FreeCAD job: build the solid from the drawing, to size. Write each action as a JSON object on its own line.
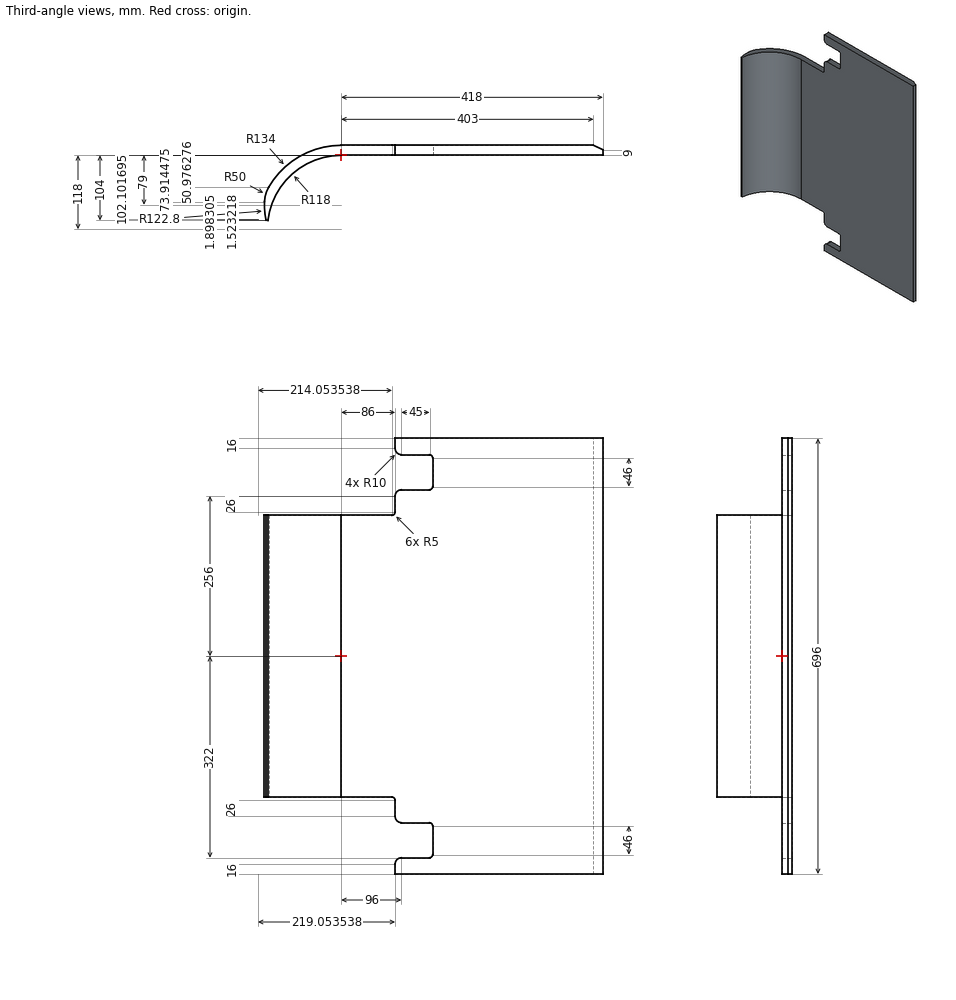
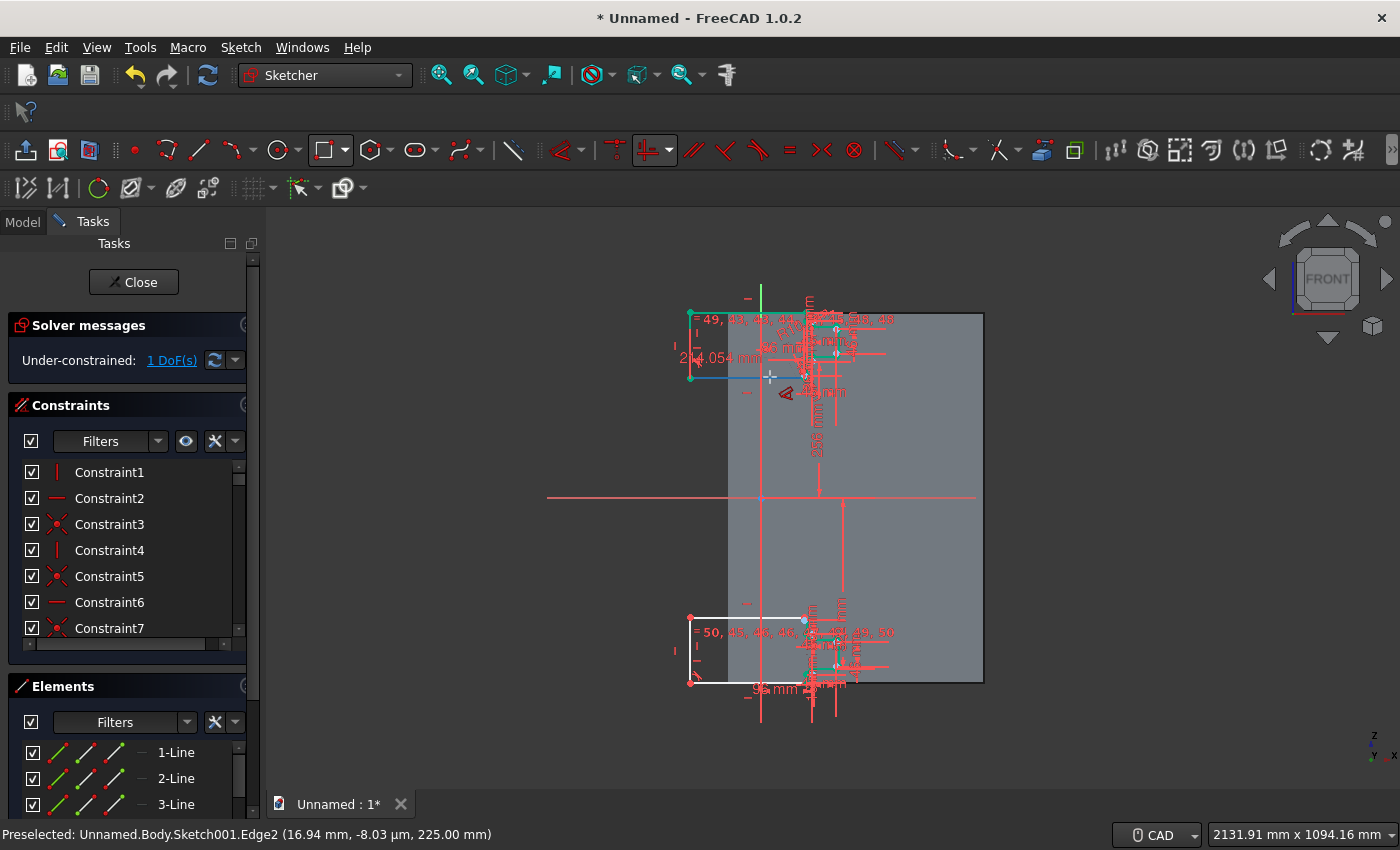
{"action": "scroll", "coordinate": [772, 683], "scroll_direction": "up", "scroll_amount": 2}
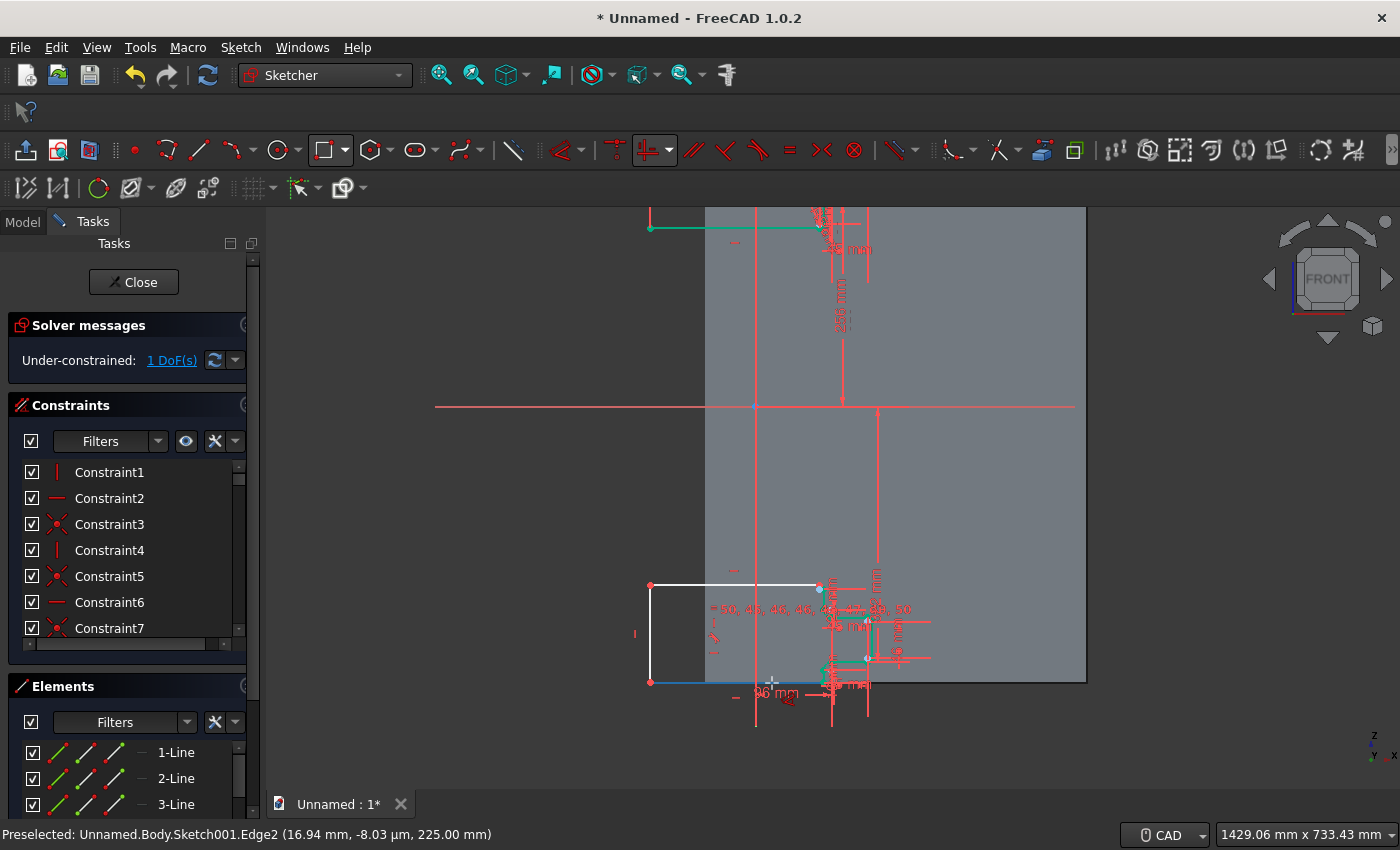
{"action": "left_click", "coordinate": [772, 683]}
{"action": "left_click", "coordinate": [737, 717]}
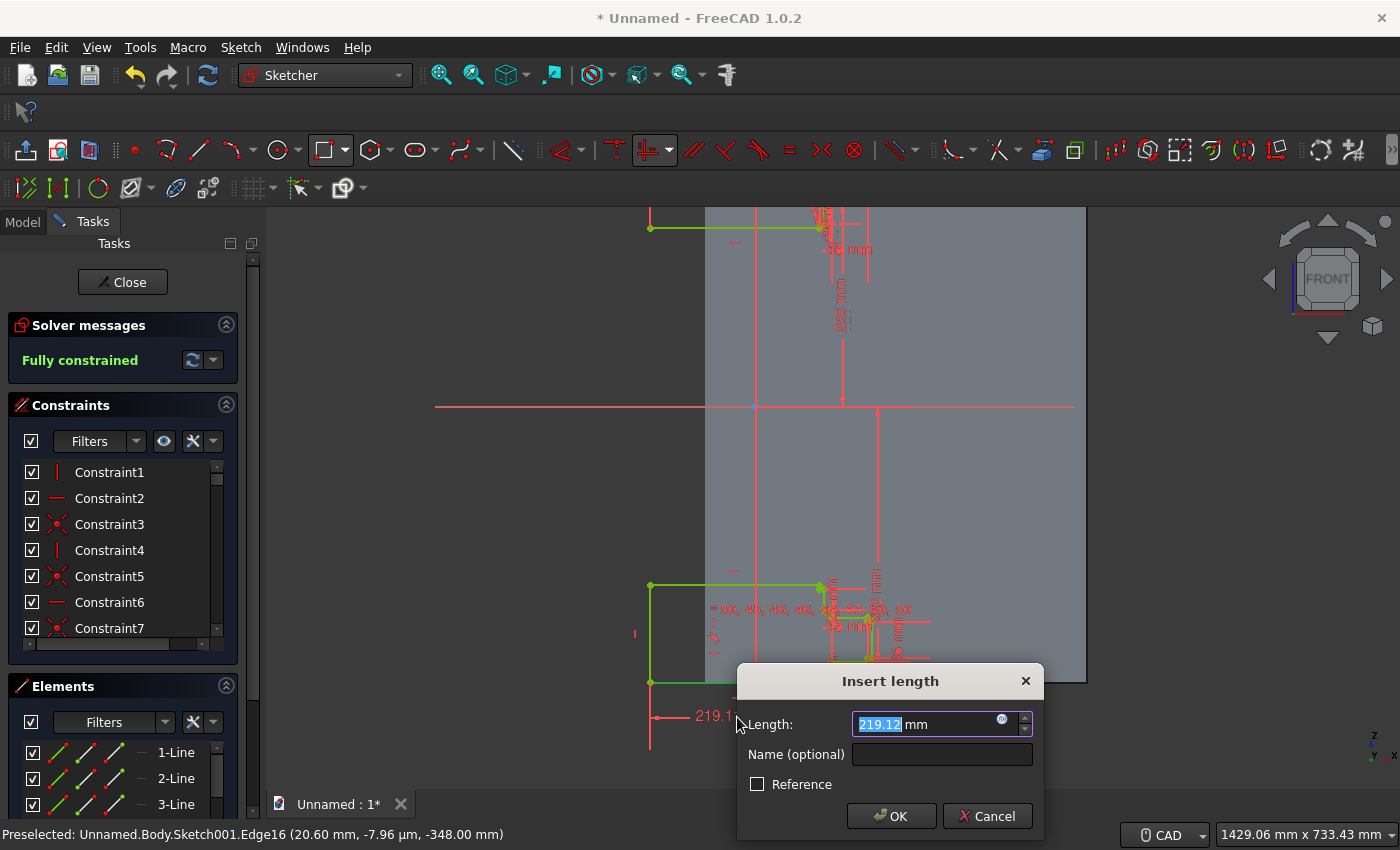
{"action": "type", "text": "219.053538"}
{"action": "key", "text": "Return"}
{"action": "key", "text": "Escape"}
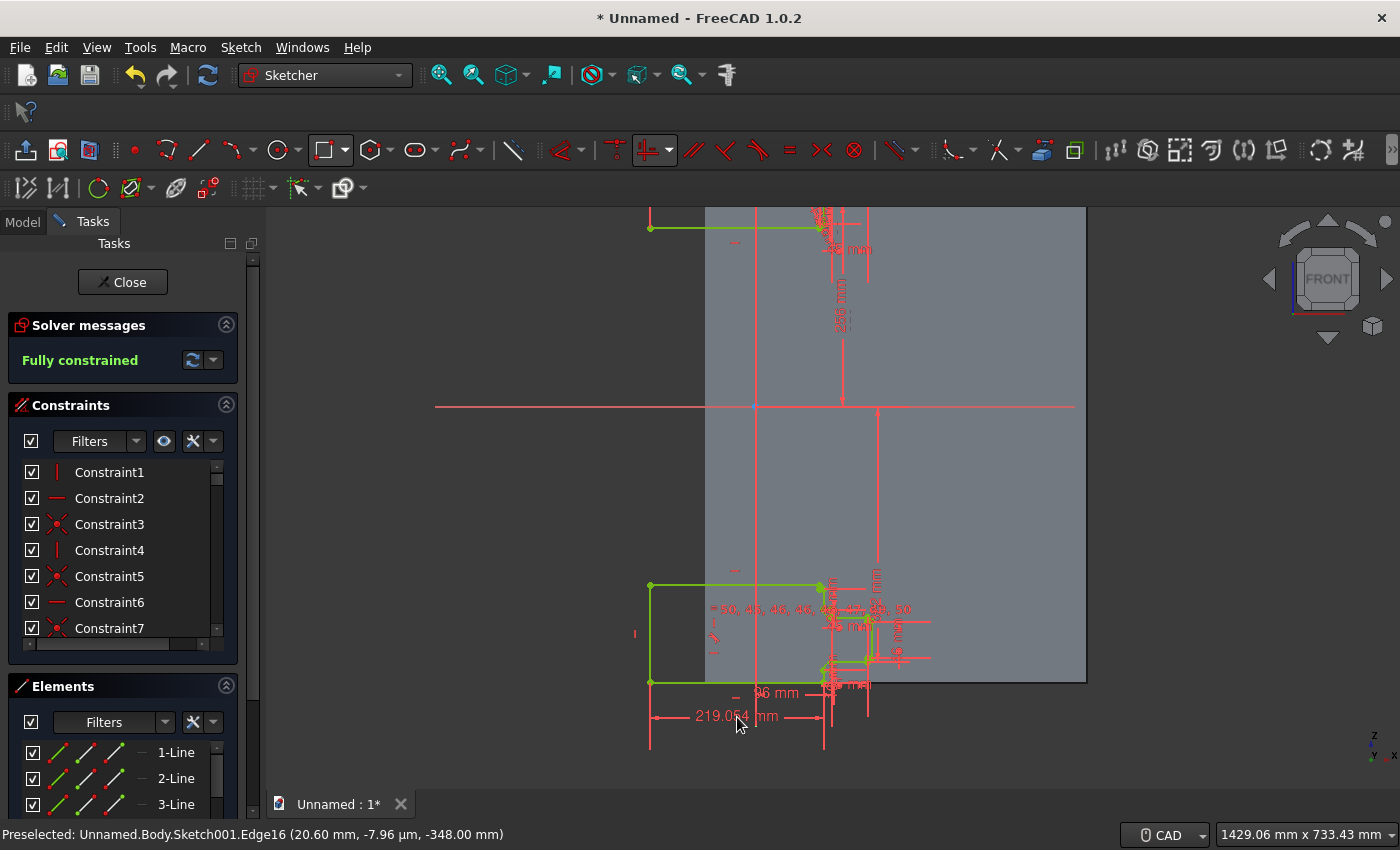
{"action": "left_click", "coordinate": [123, 282]}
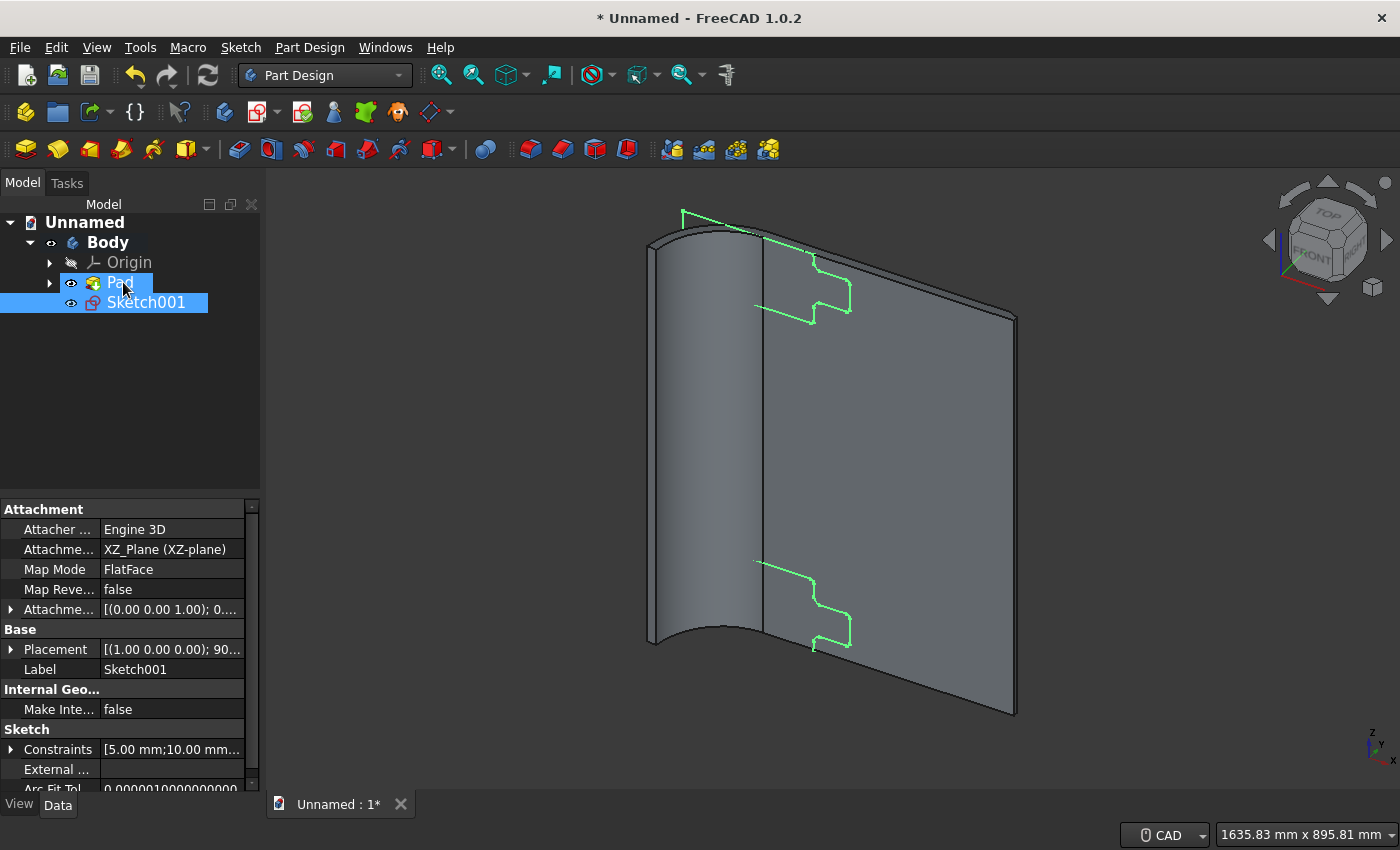
{"action": "left_click", "coordinate": [240, 150]}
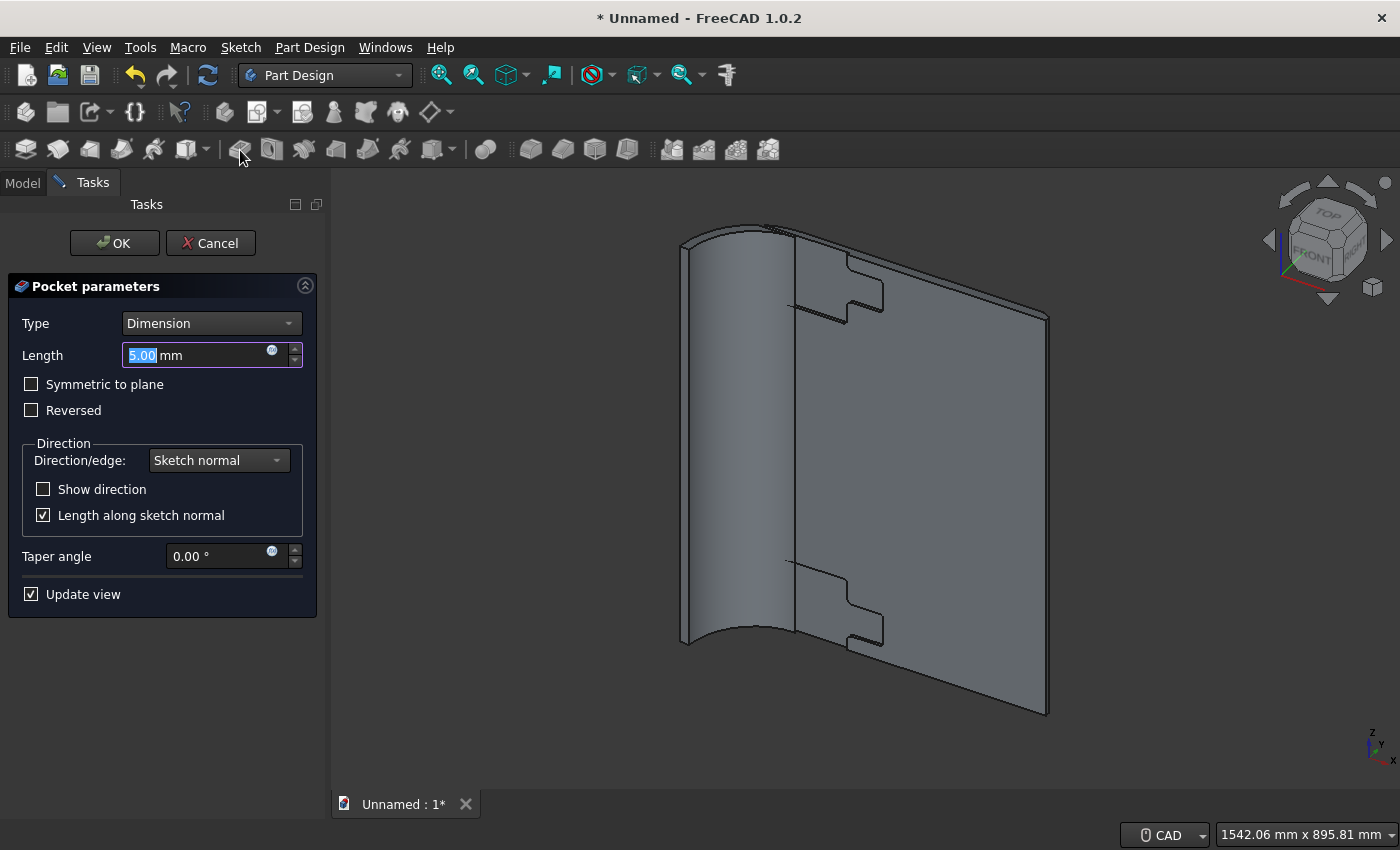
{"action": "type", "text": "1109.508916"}
{"action": "key", "text": "Tab"}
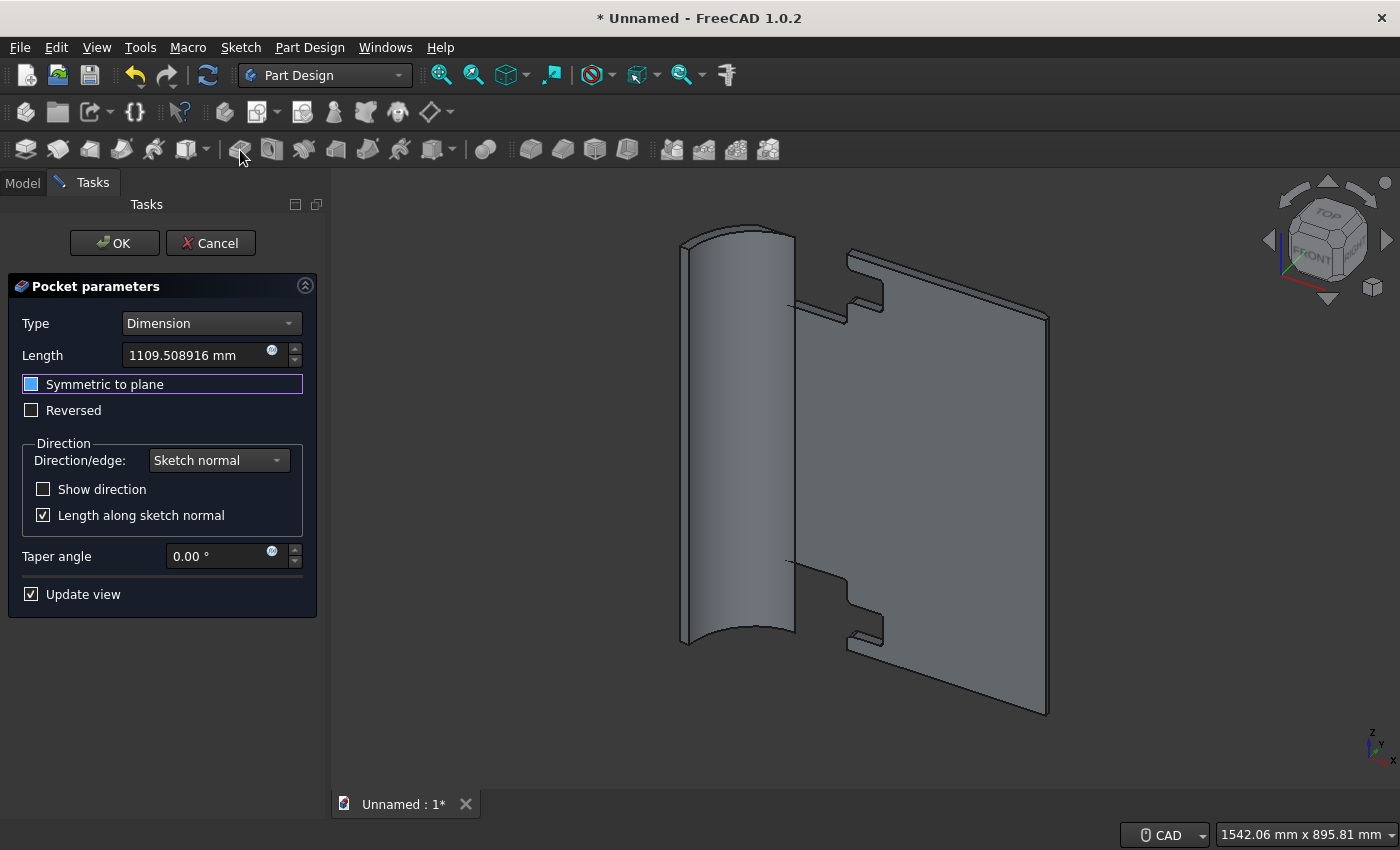
{"action": "left_click", "coordinate": [30, 384]}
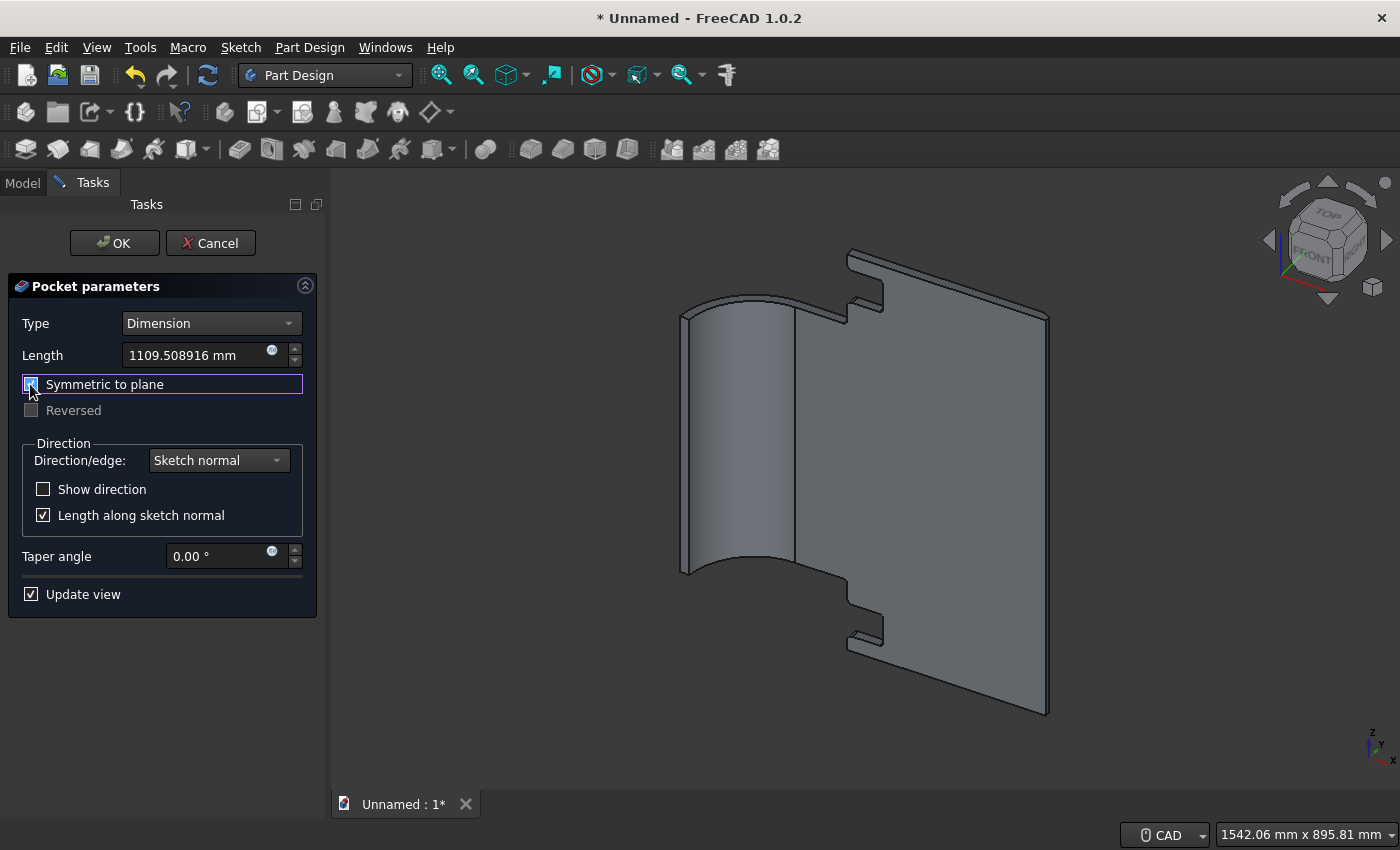
{"action": "left_click", "coordinate": [115, 243]}